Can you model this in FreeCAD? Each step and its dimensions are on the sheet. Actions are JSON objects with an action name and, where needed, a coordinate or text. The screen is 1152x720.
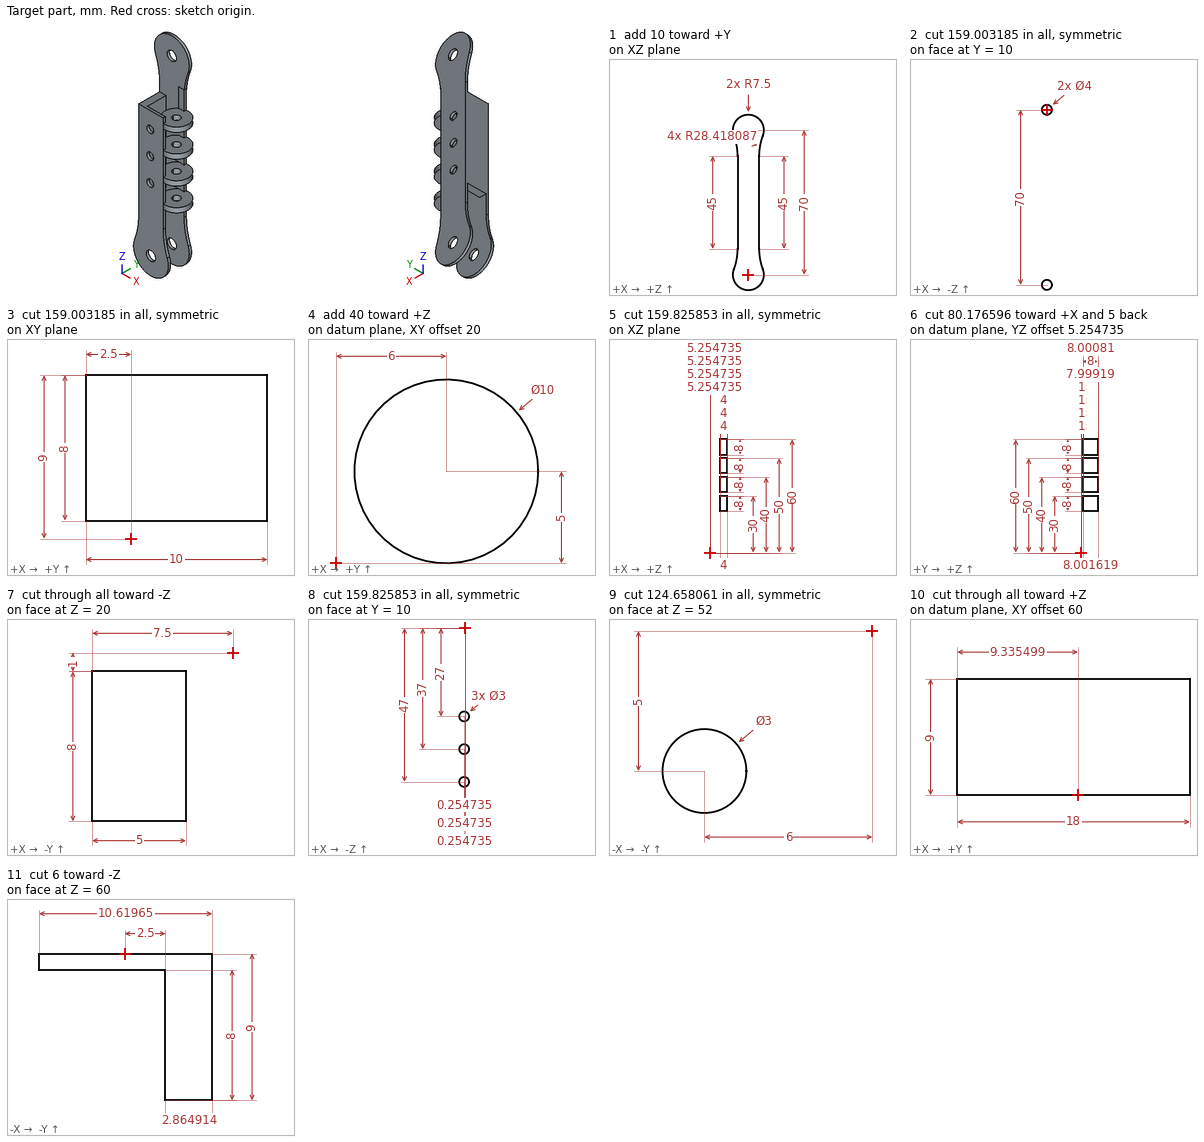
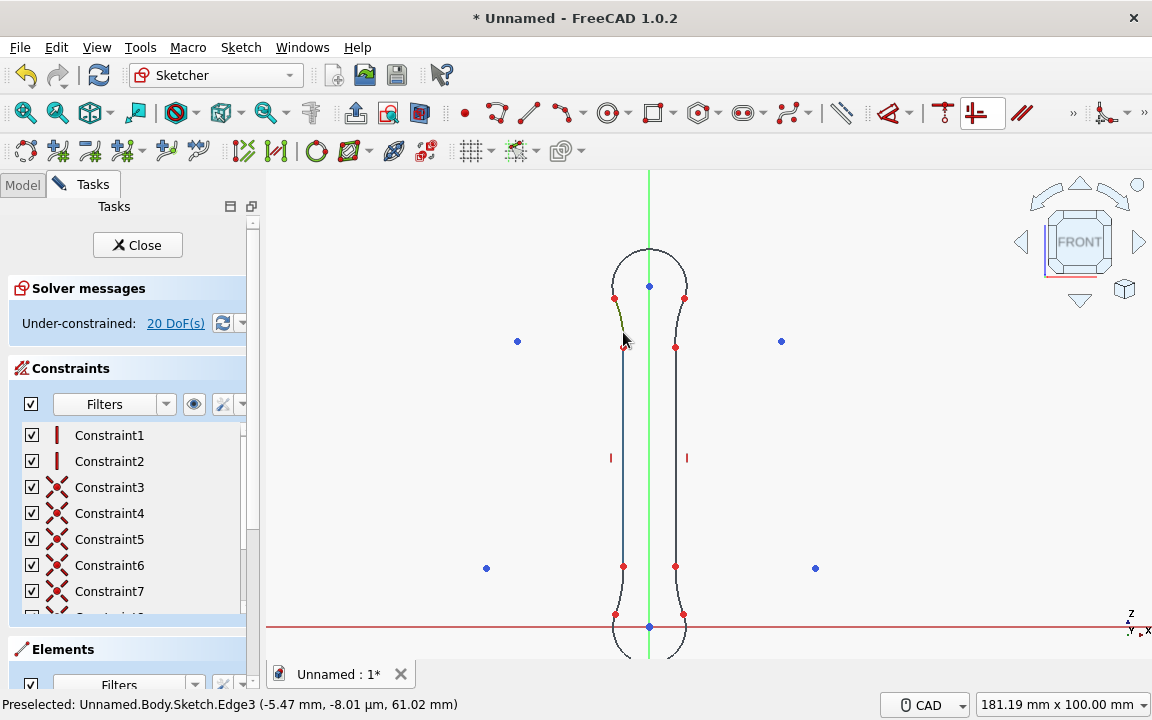
{"action": "key", "text": "t"}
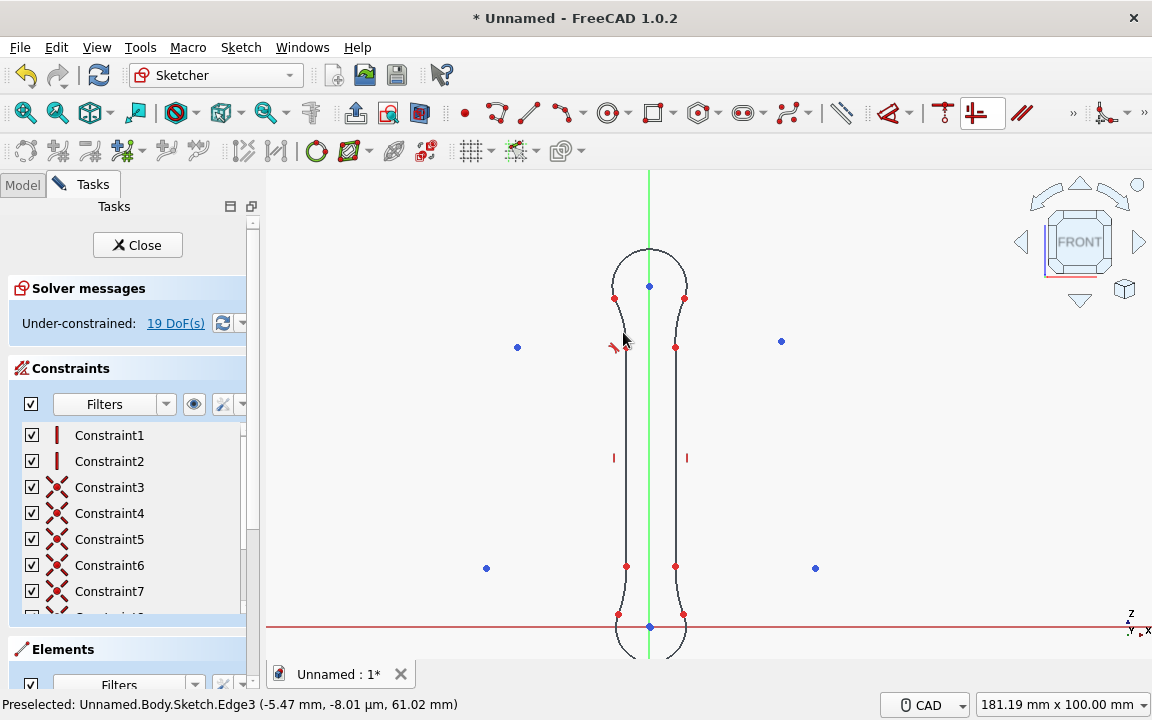
{"action": "left_click", "coordinate": [626, 501]}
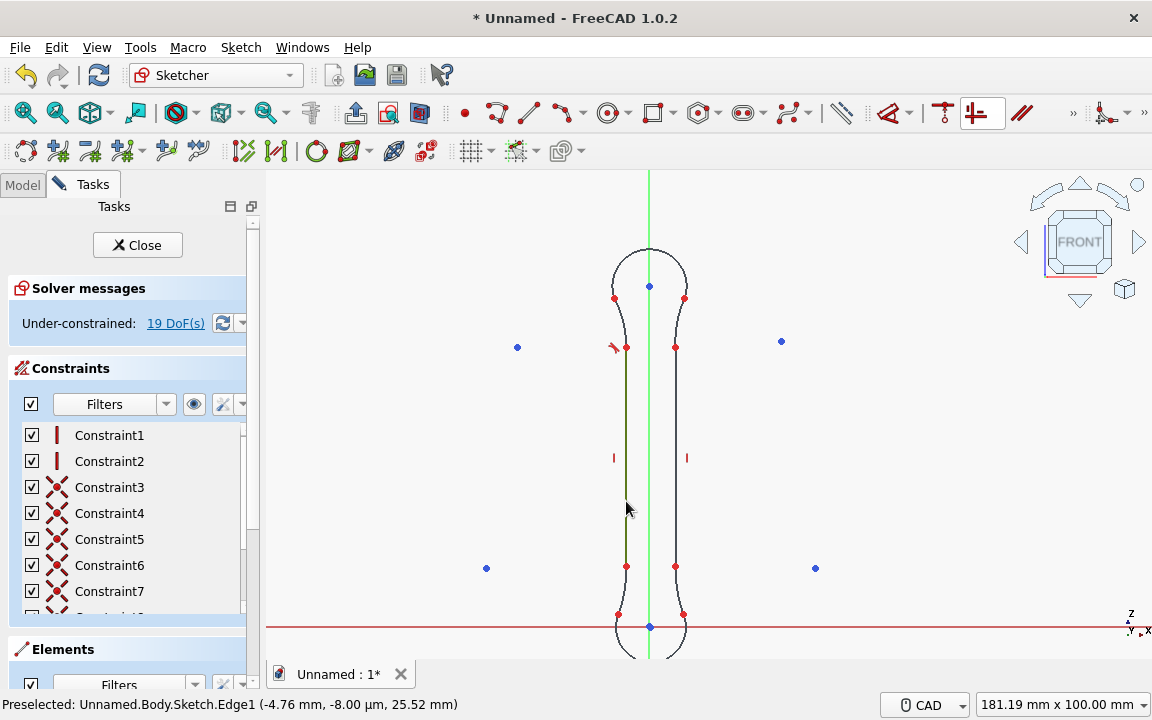
{"action": "left_click", "coordinate": [623, 601]}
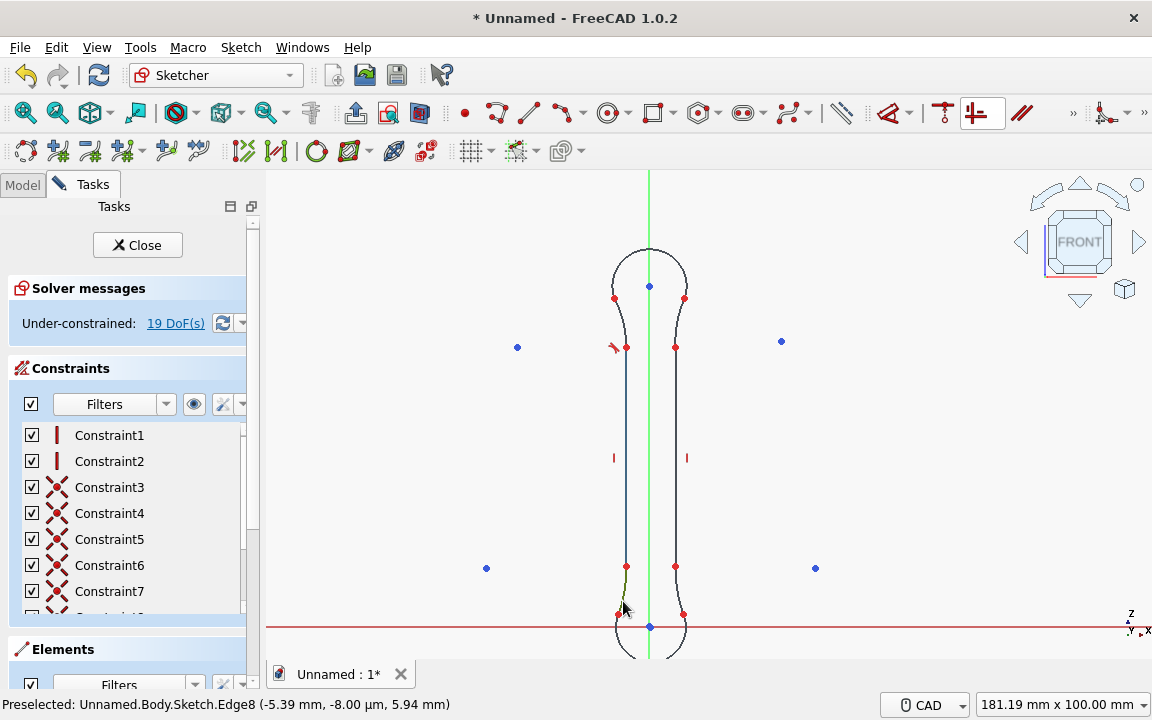
{"action": "key", "text": "t"}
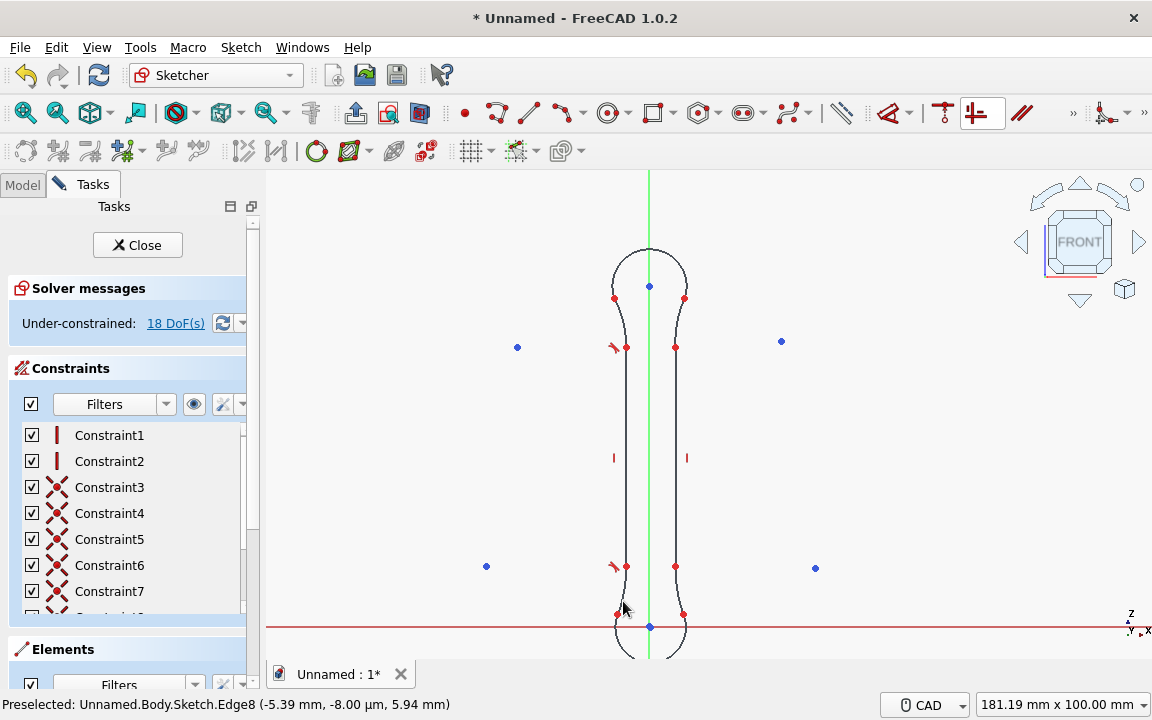
{"action": "left_click", "coordinate": [676, 413]}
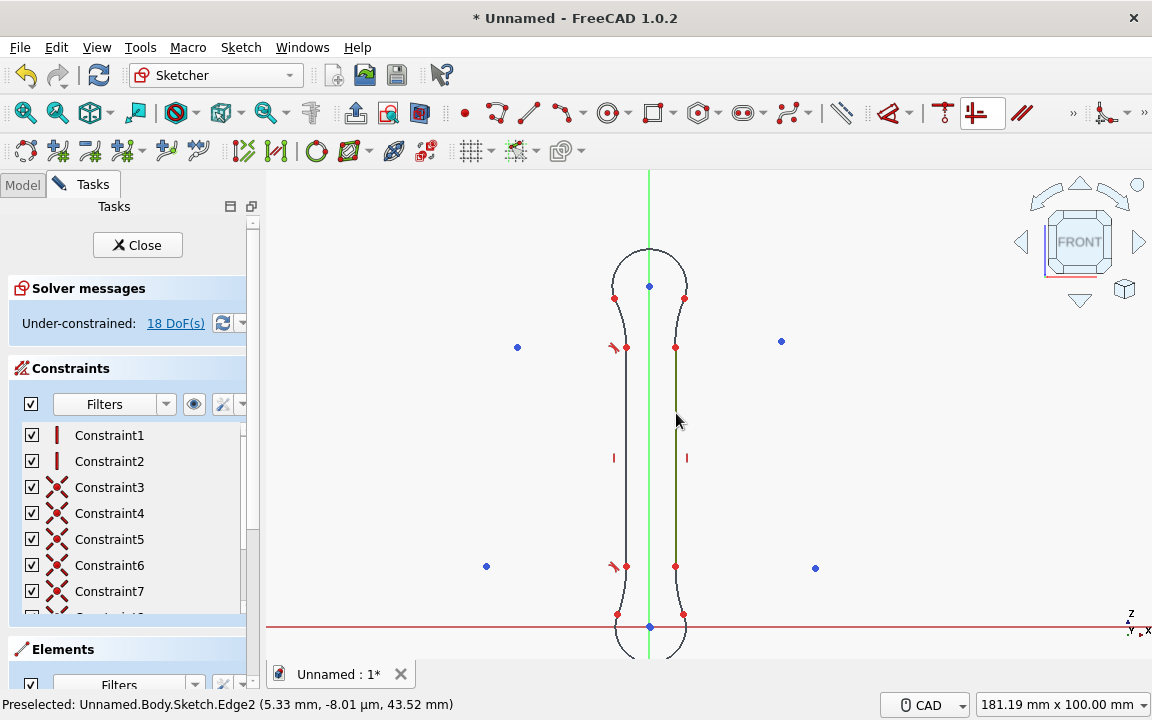
{"action": "left_click", "coordinate": [679, 313]}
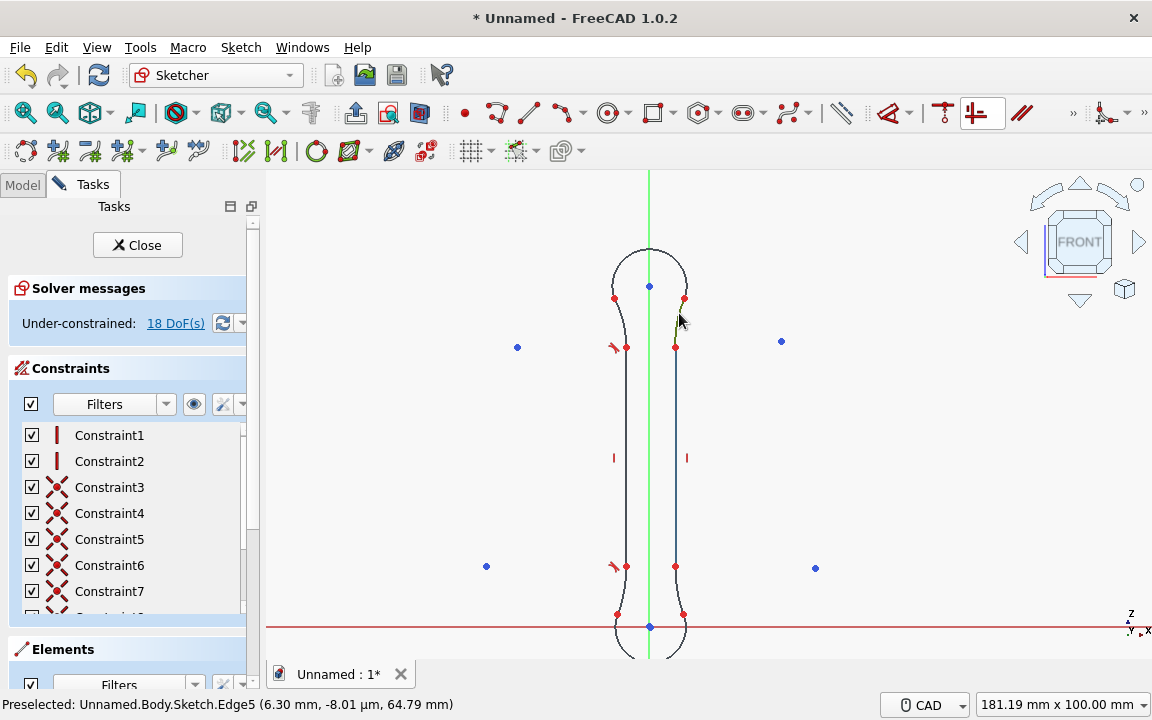
{"action": "key", "text": "t"}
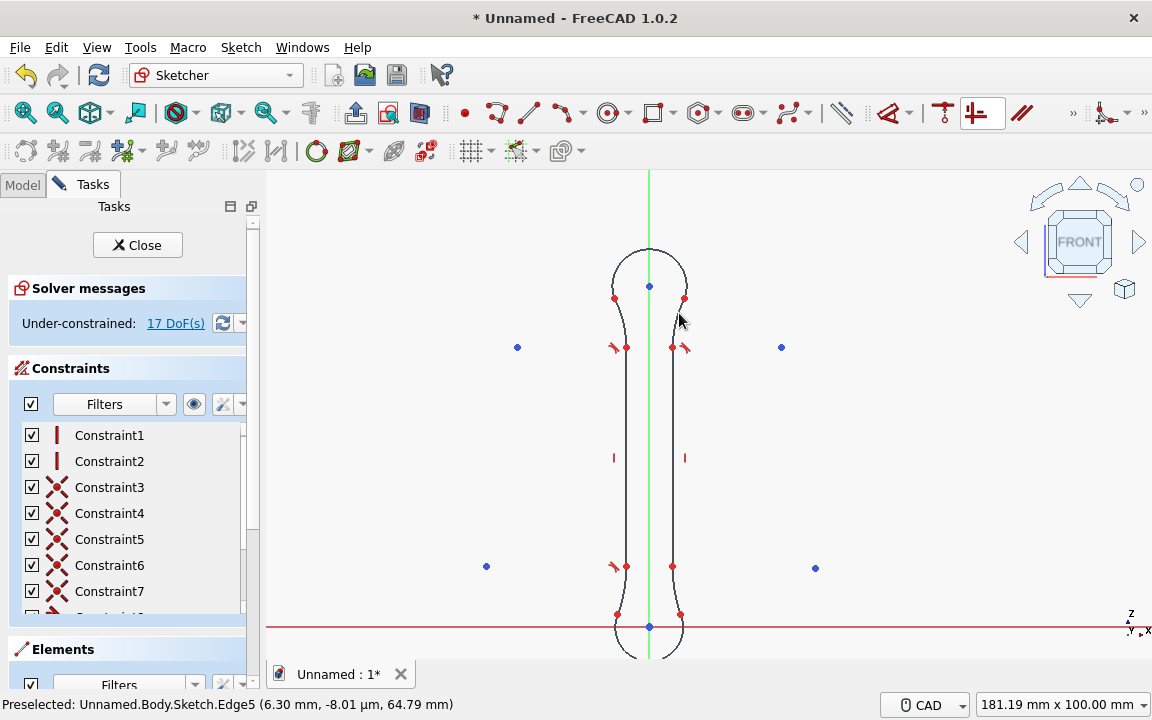
{"action": "left_click", "coordinate": [673, 413]}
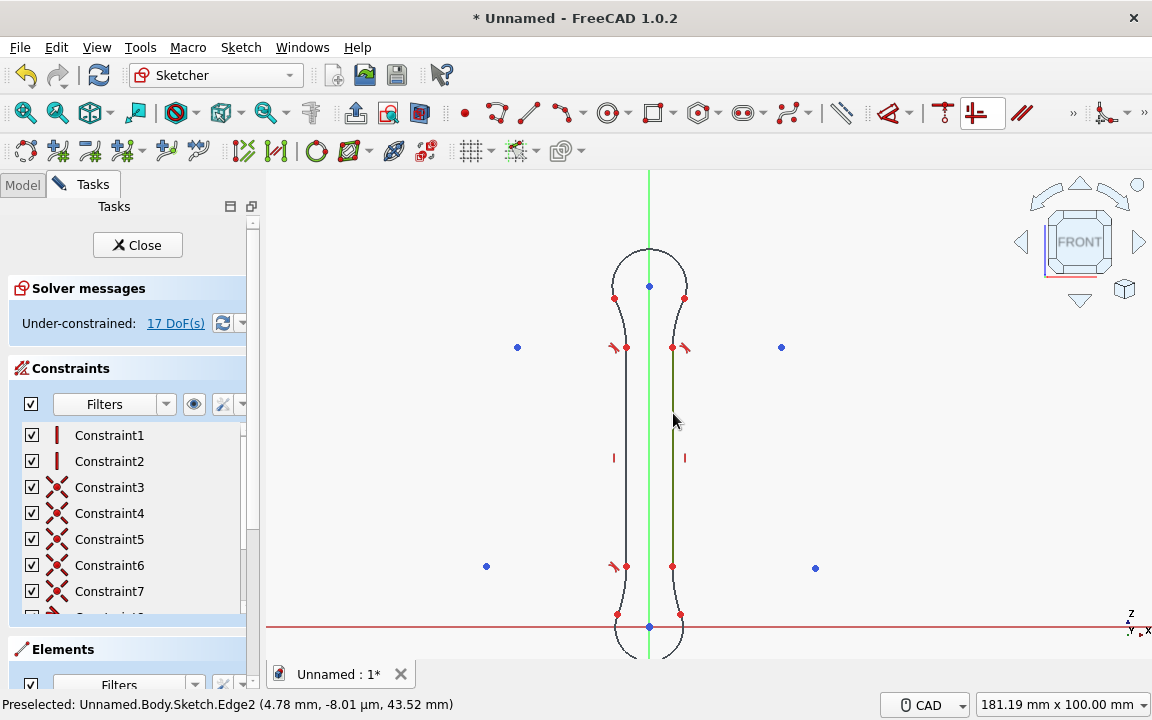
{"action": "left_click", "coordinate": [673, 581]}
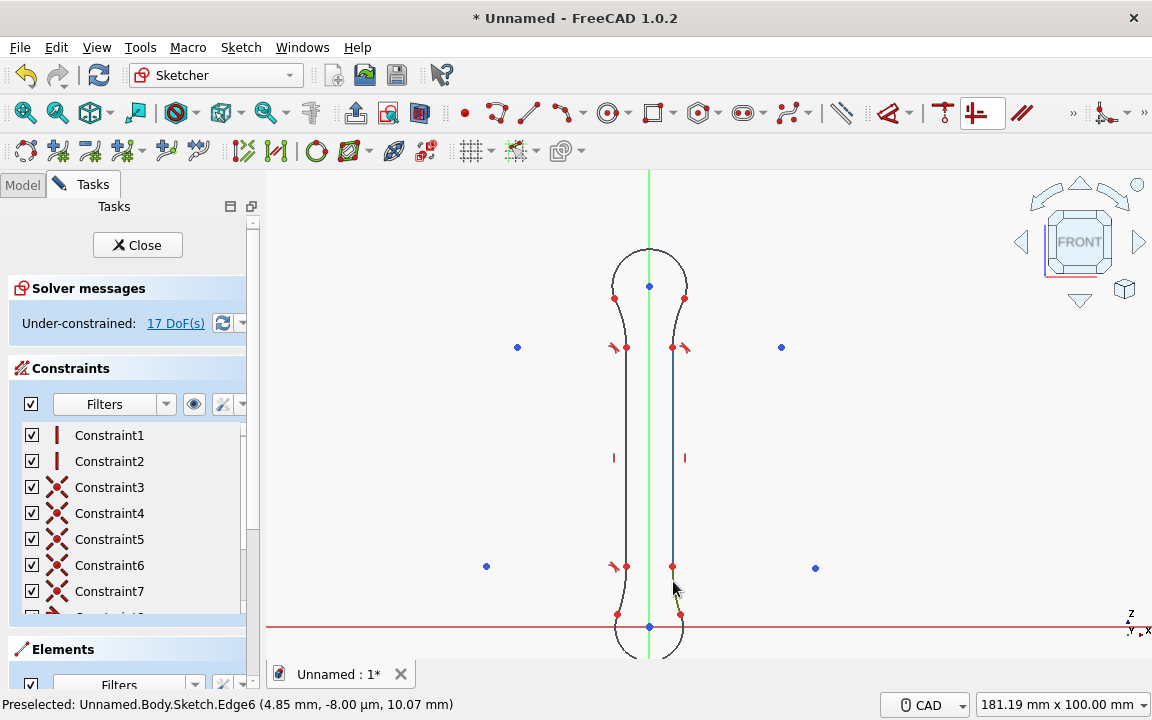
{"action": "key", "text": "t"}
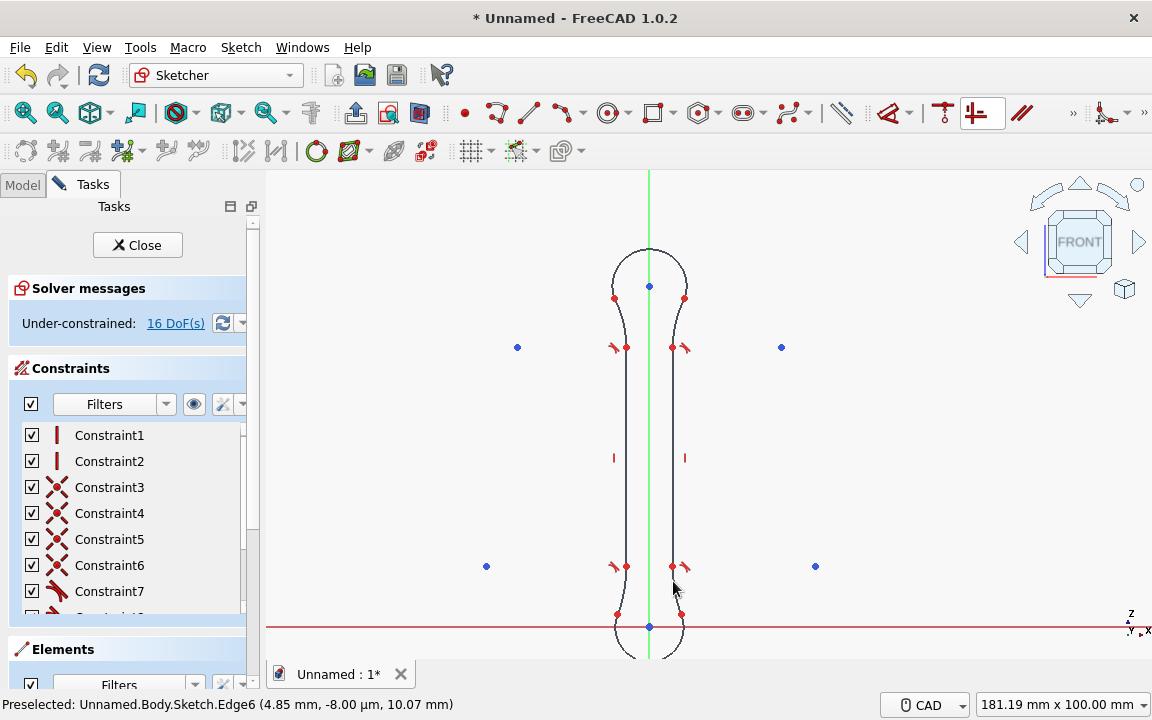
{"action": "left_click", "coordinate": [625, 332]}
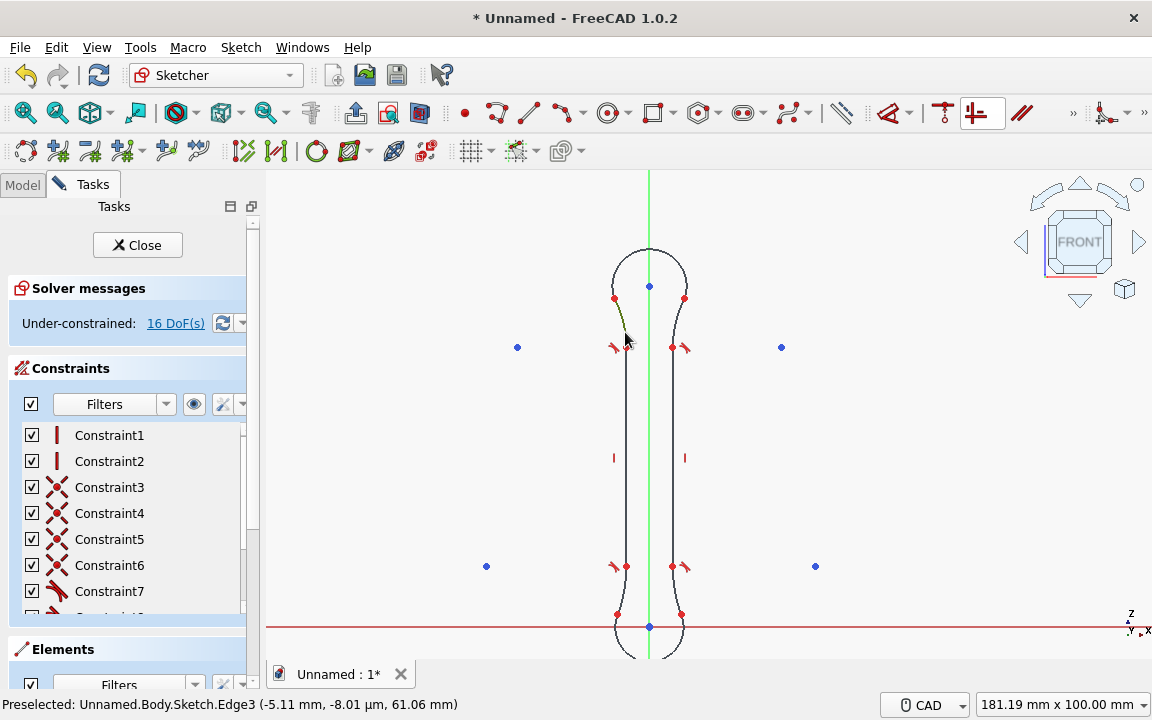
{"action": "left_click", "coordinate": [675, 260]}